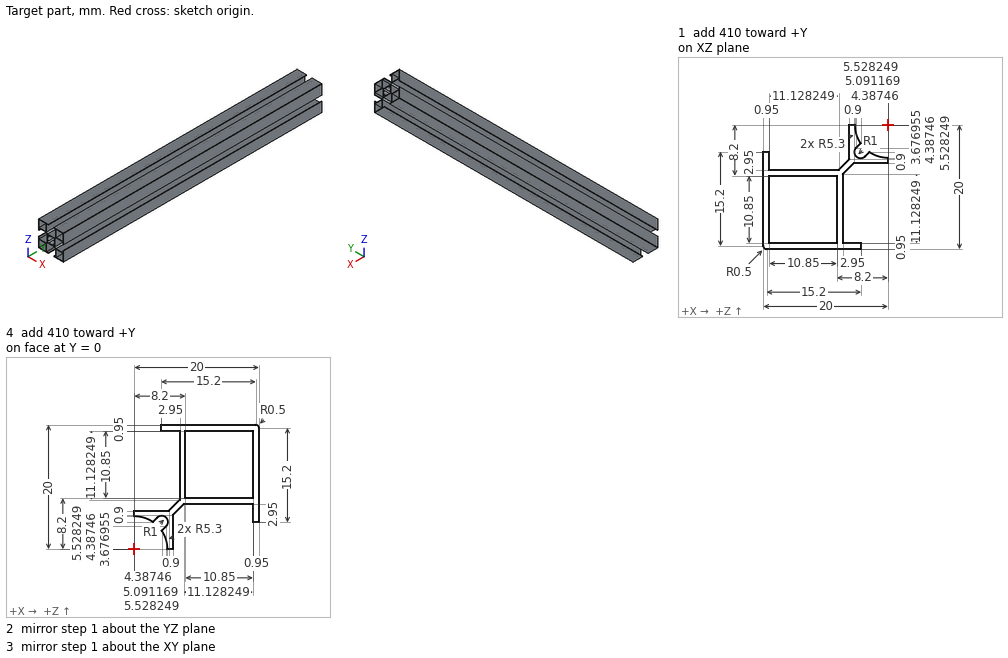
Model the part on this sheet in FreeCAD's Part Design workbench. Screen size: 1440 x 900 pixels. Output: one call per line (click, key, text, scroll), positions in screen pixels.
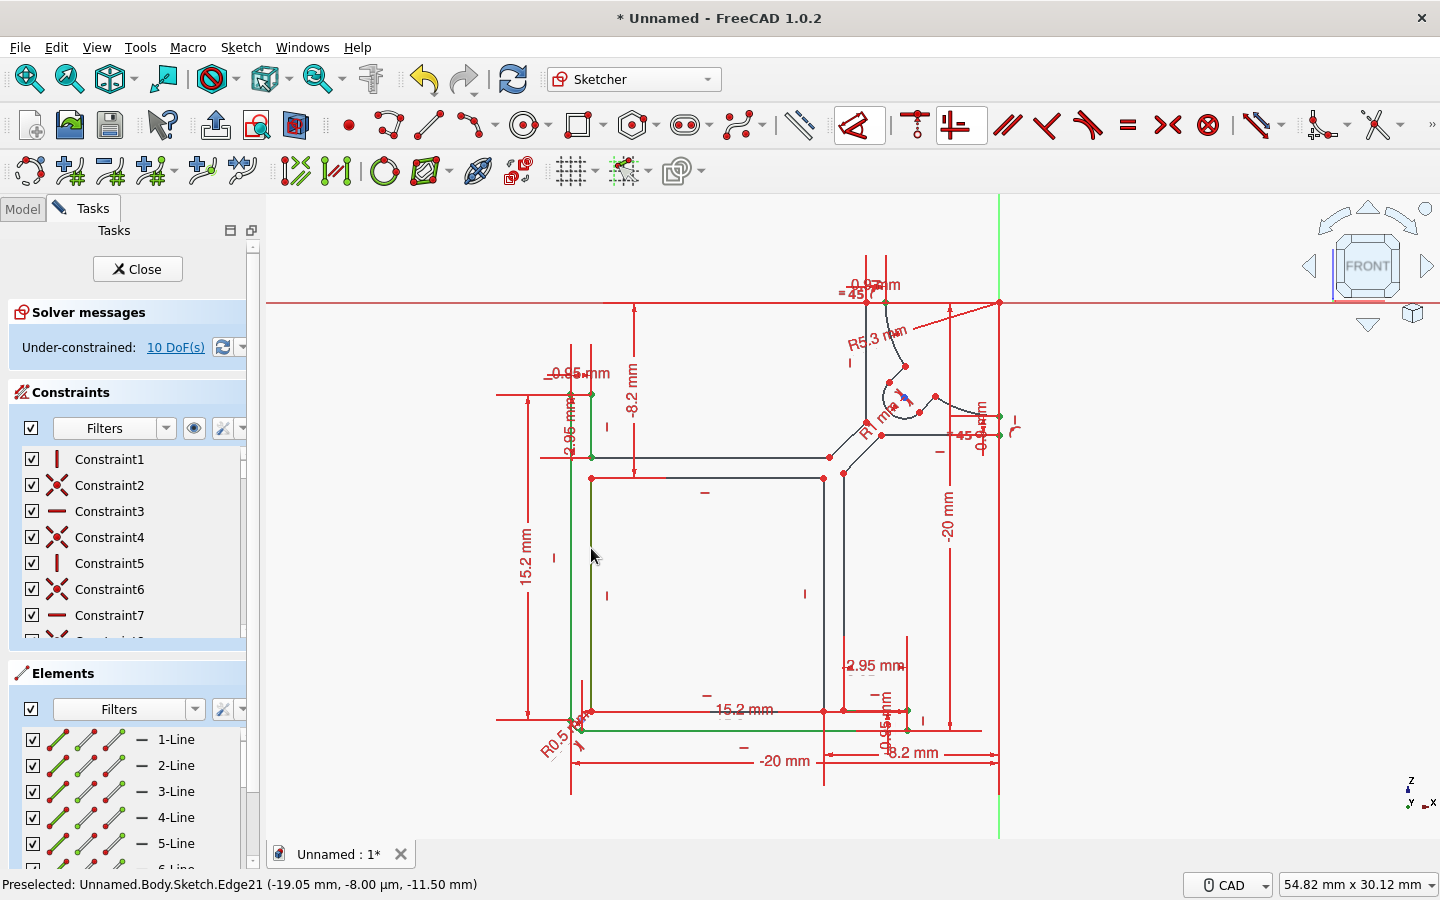
click(880, 126)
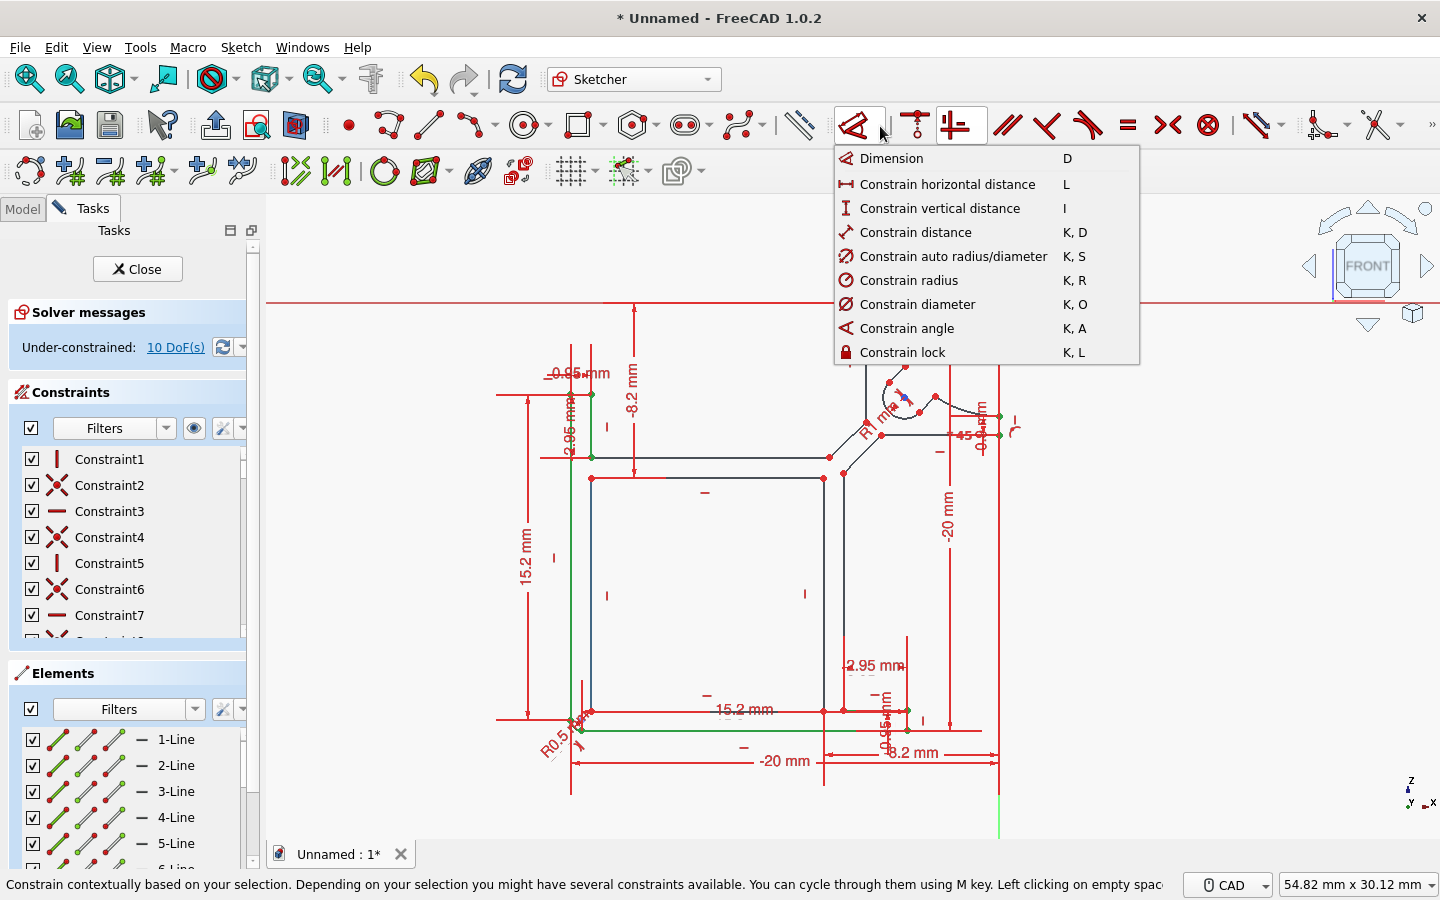
click(987, 208)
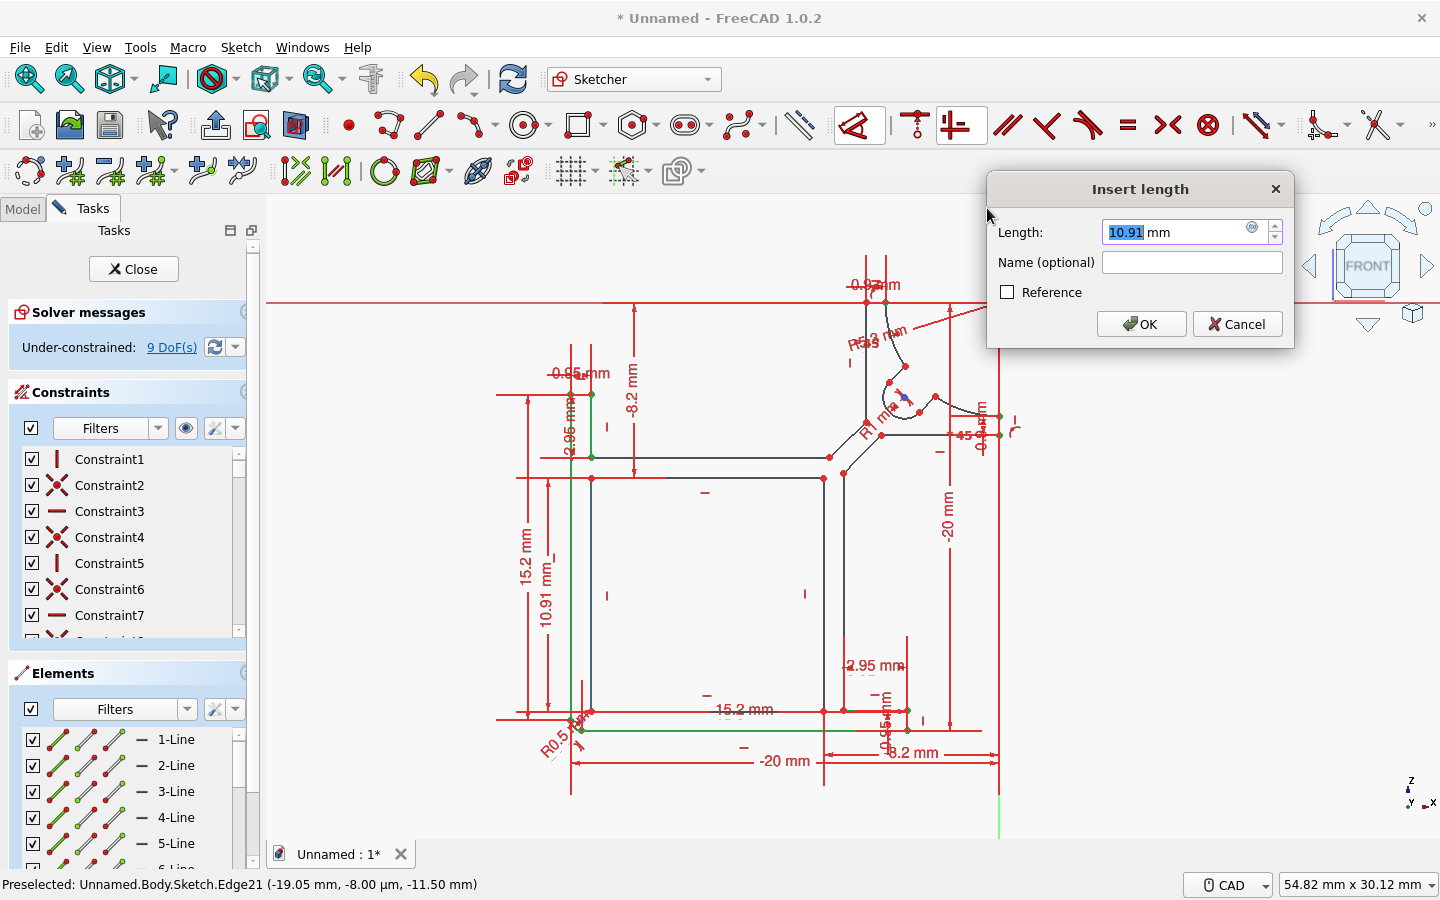
text(10.85)
key(Return)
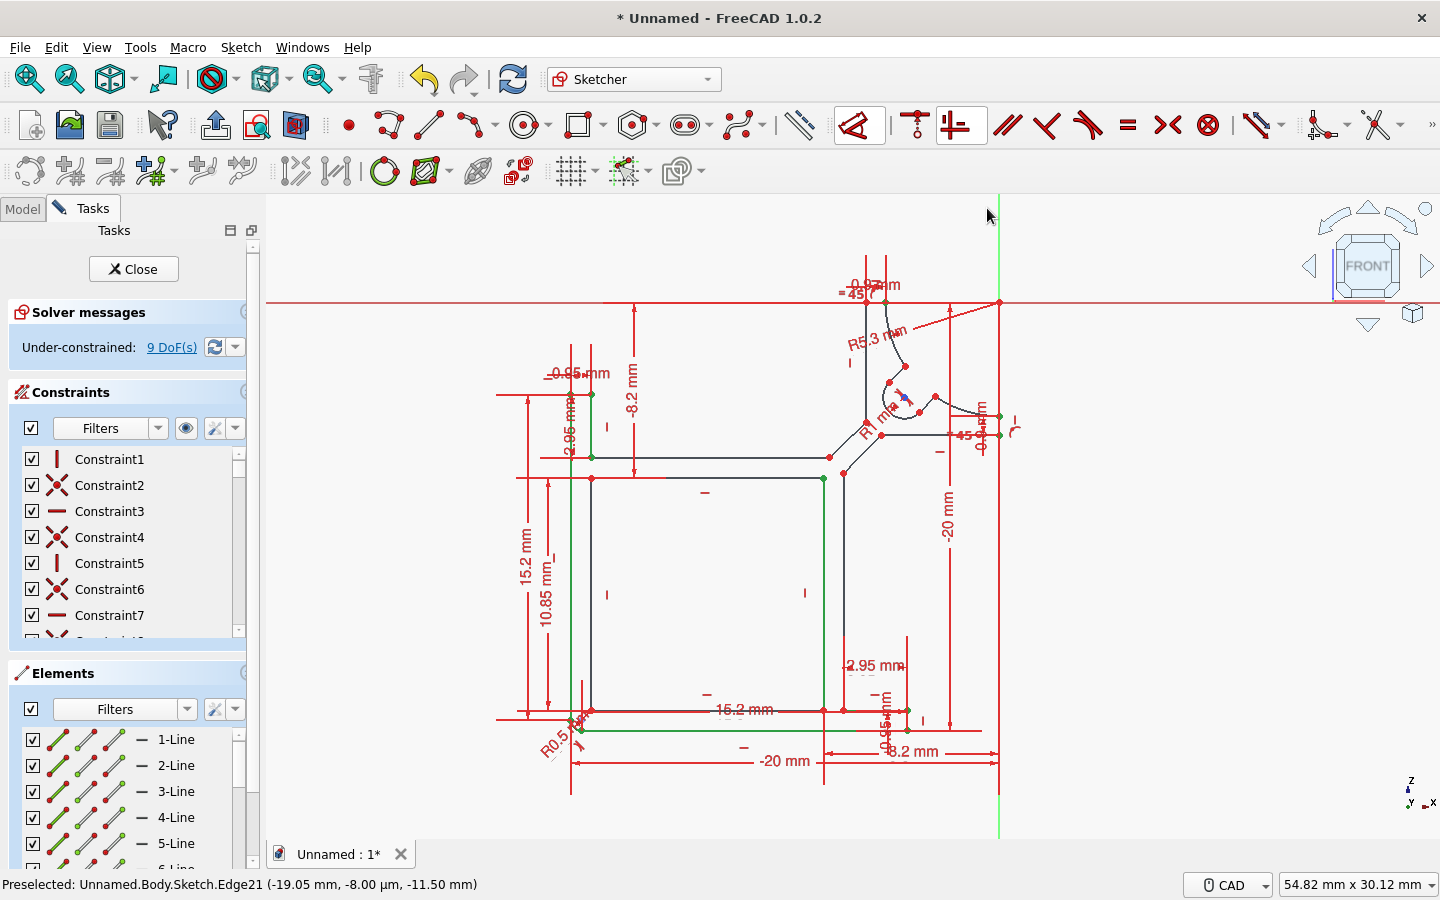
click(661, 711)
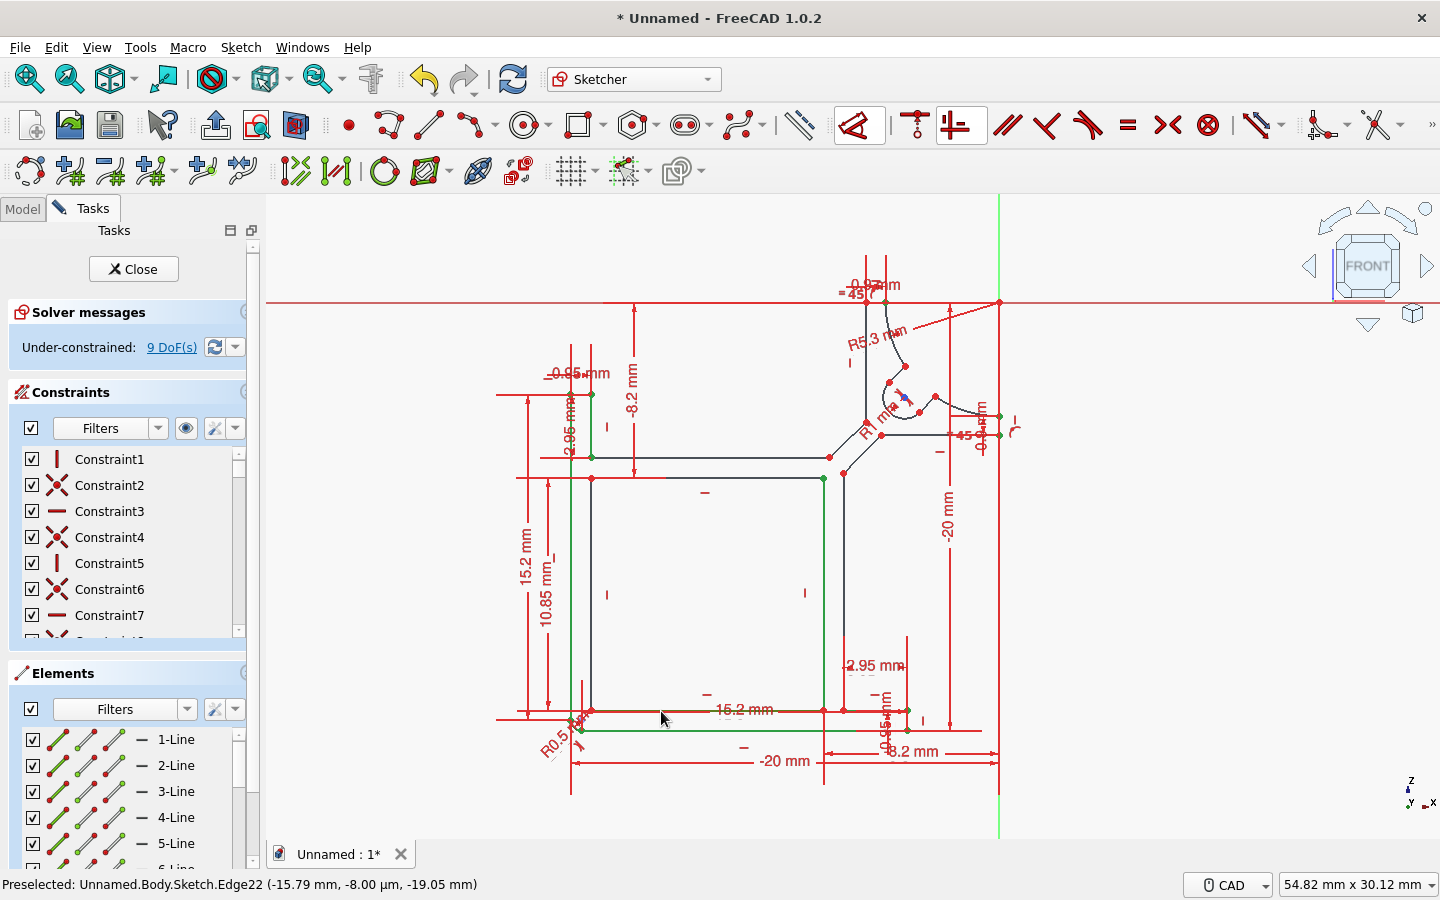
click(880, 126)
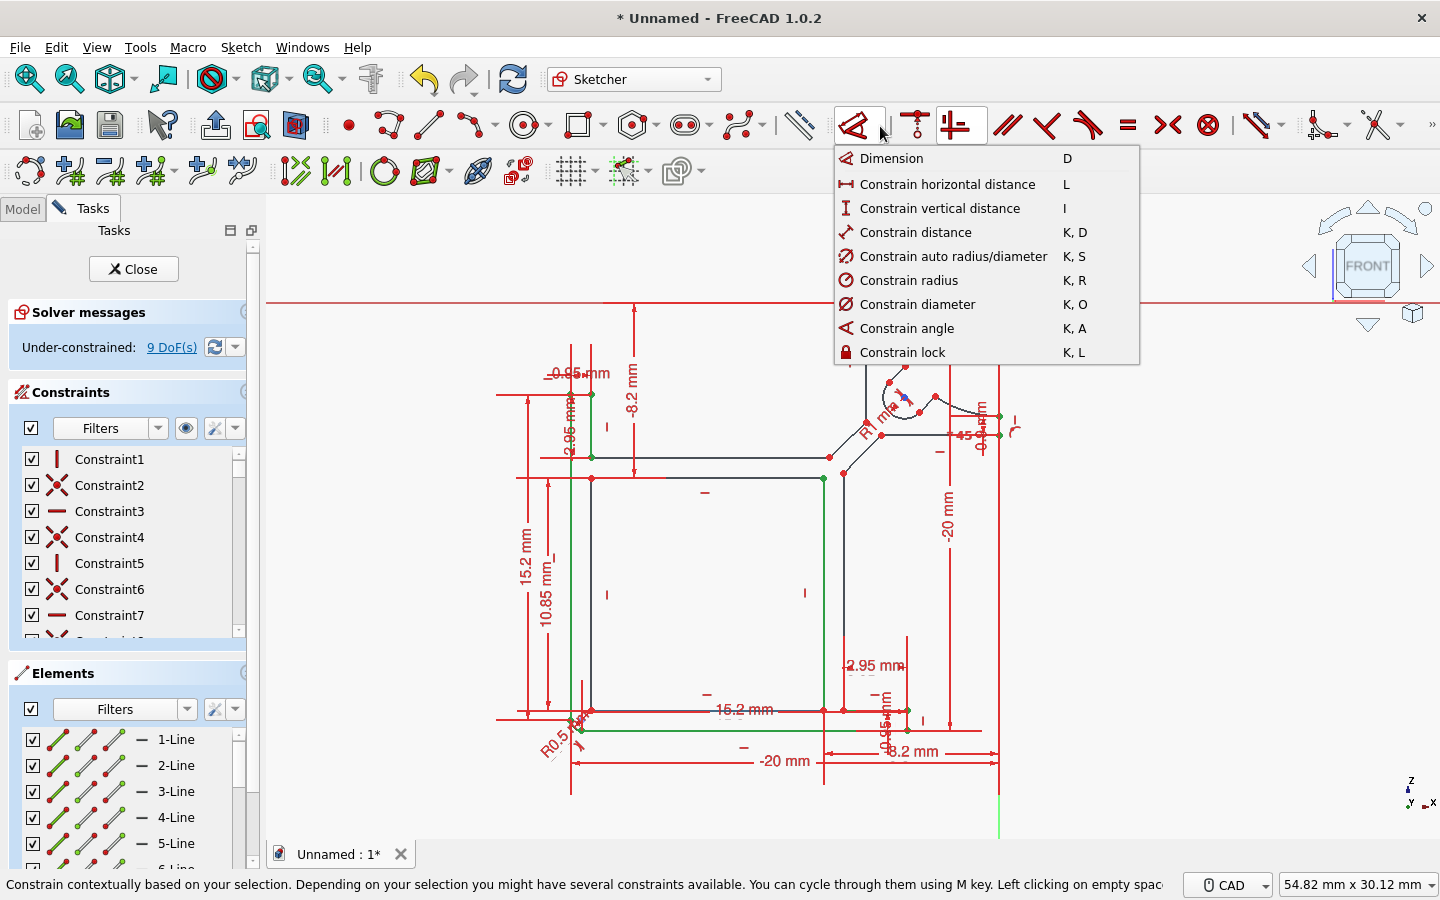
click(987, 184)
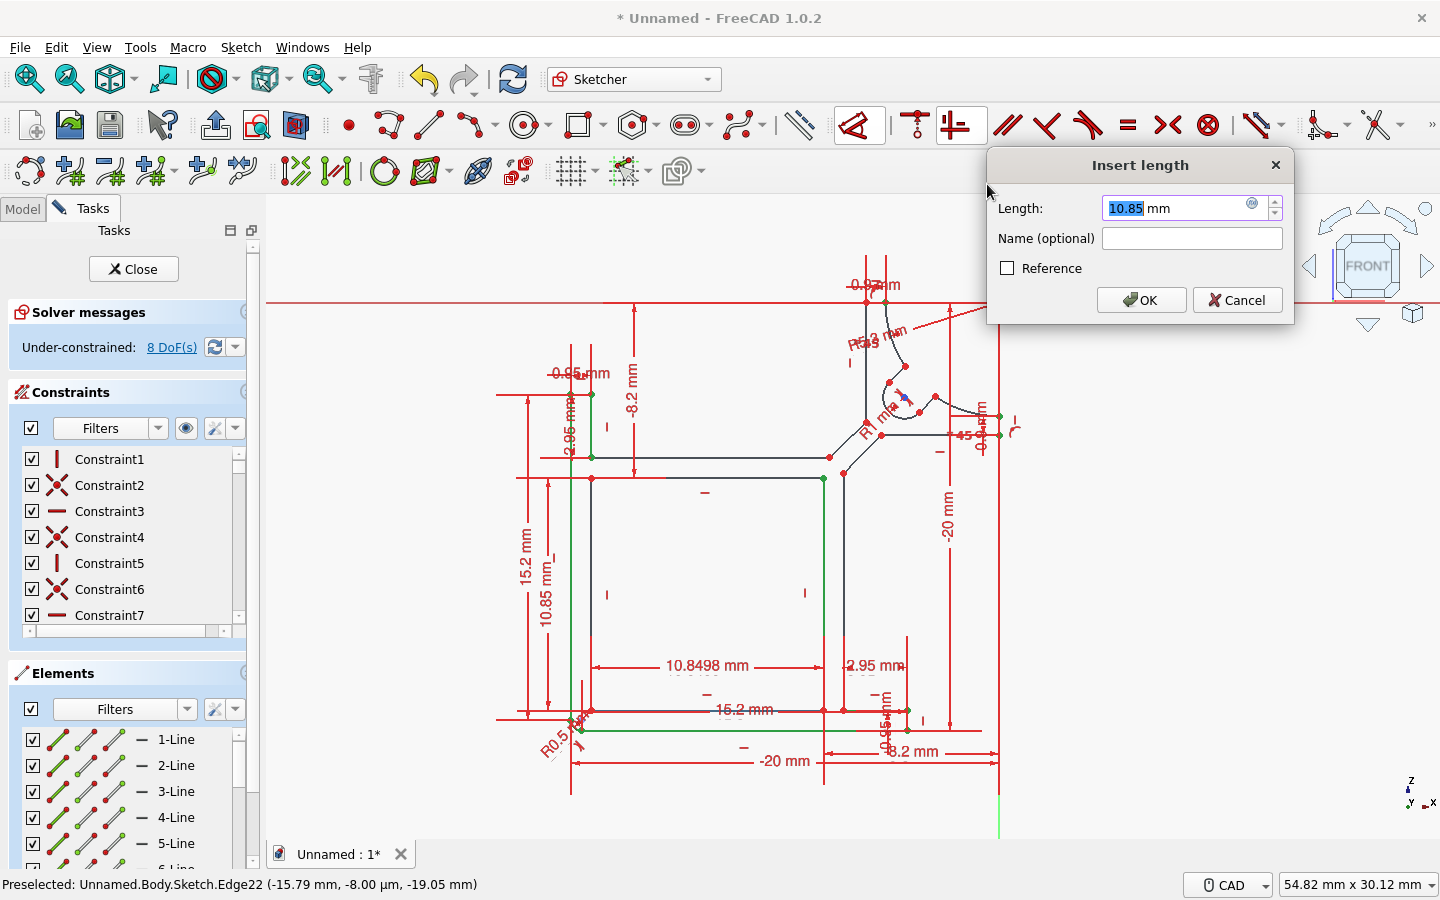
text(10.85)
key(Return)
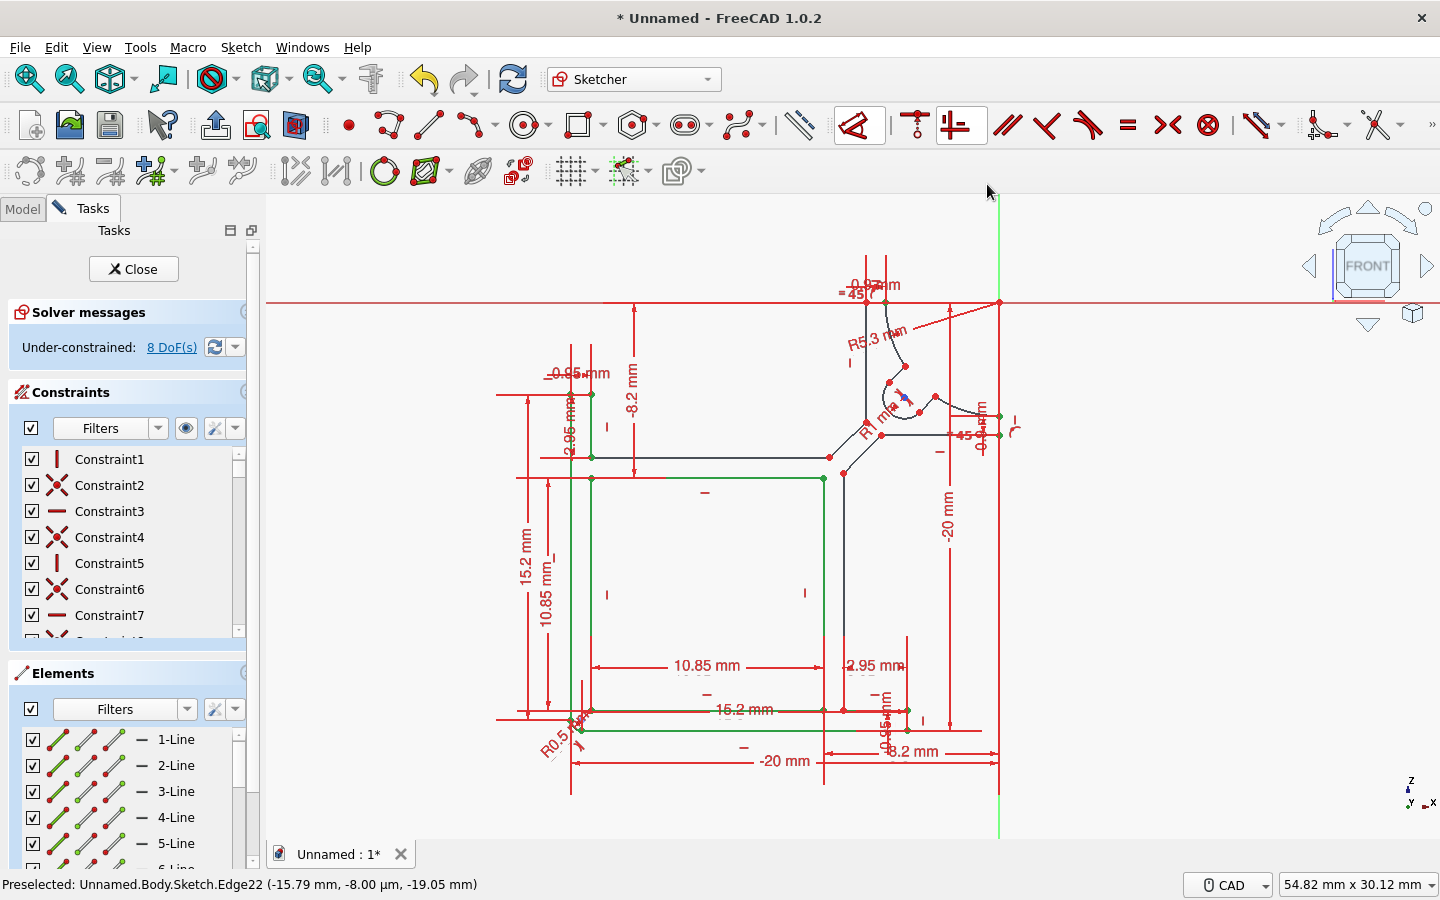
click(866, 386)